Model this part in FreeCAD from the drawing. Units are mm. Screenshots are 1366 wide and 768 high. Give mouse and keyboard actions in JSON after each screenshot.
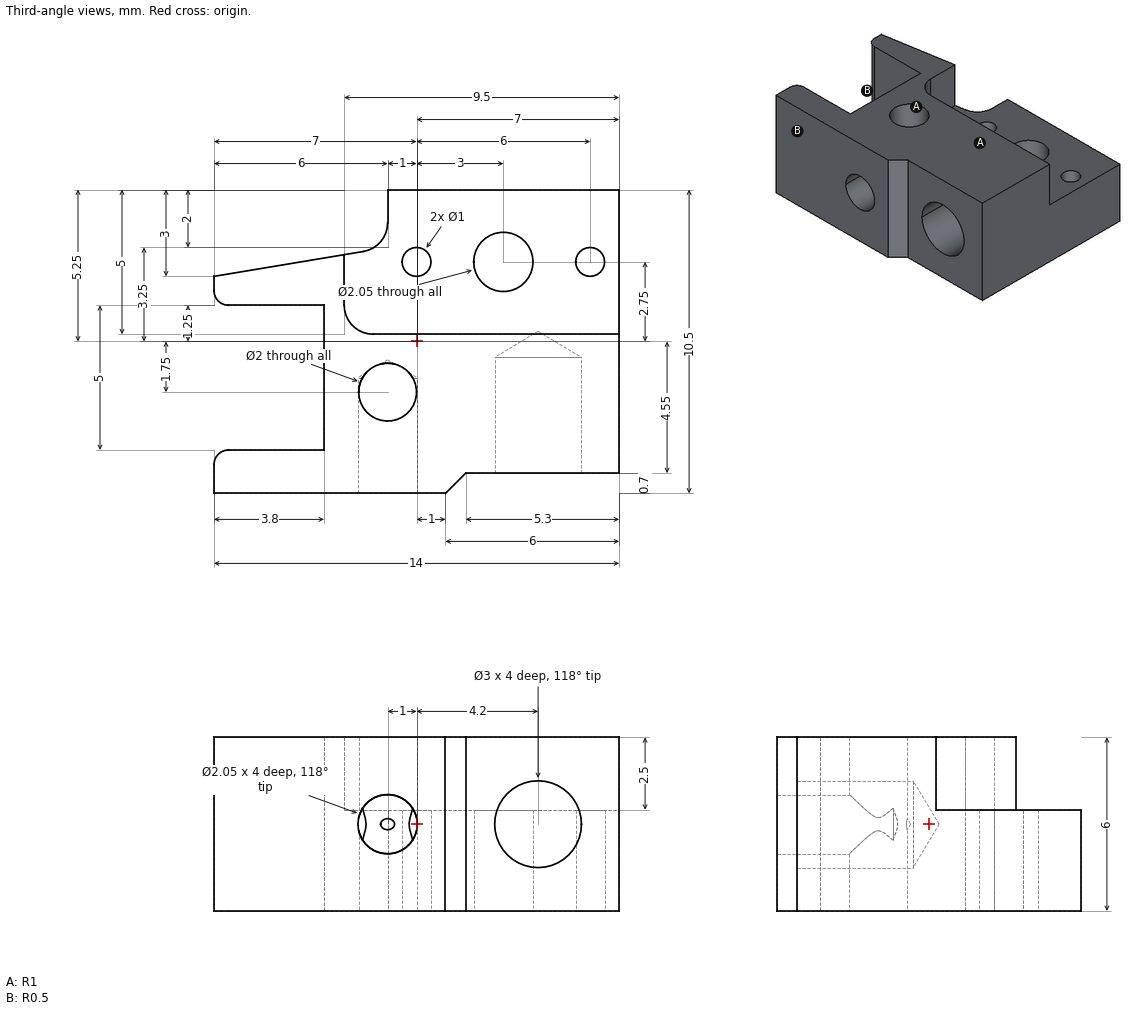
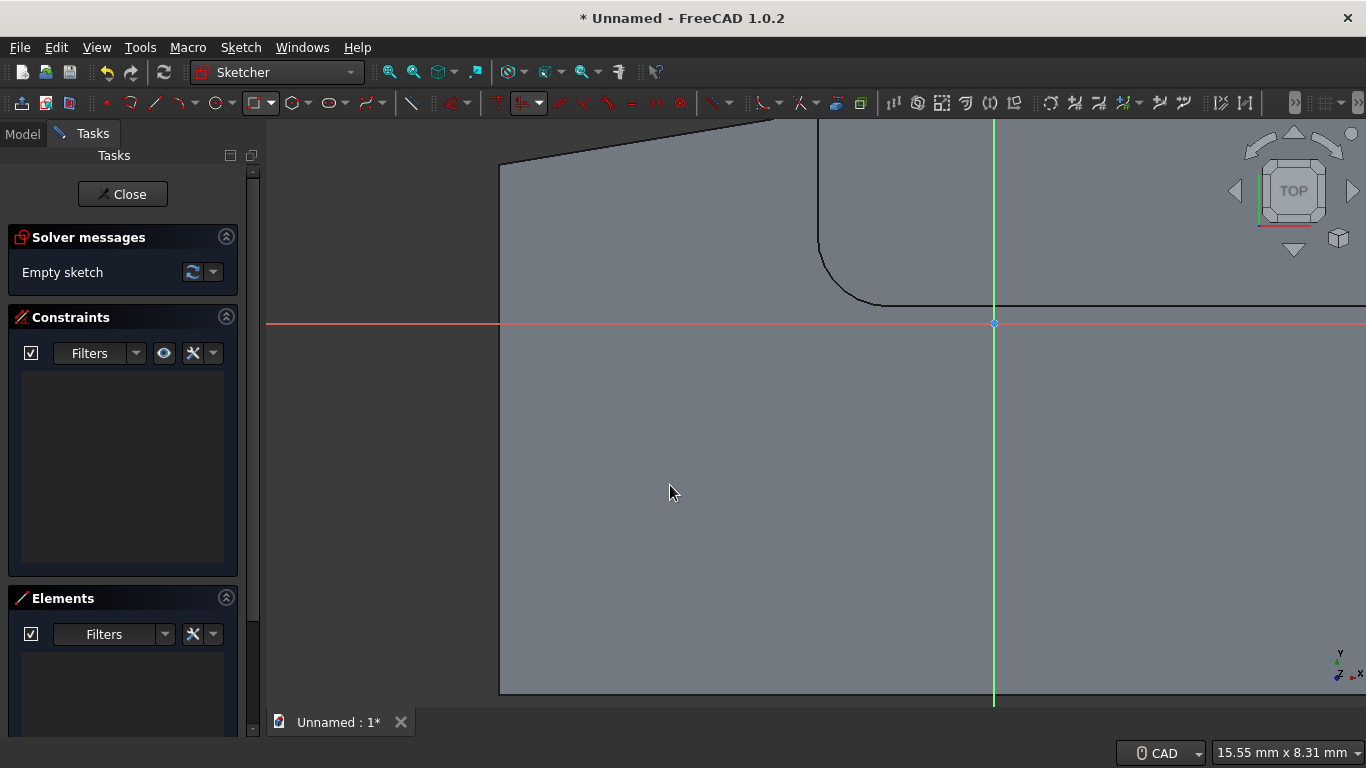
{"action": "left_click", "coordinate": [254, 104]}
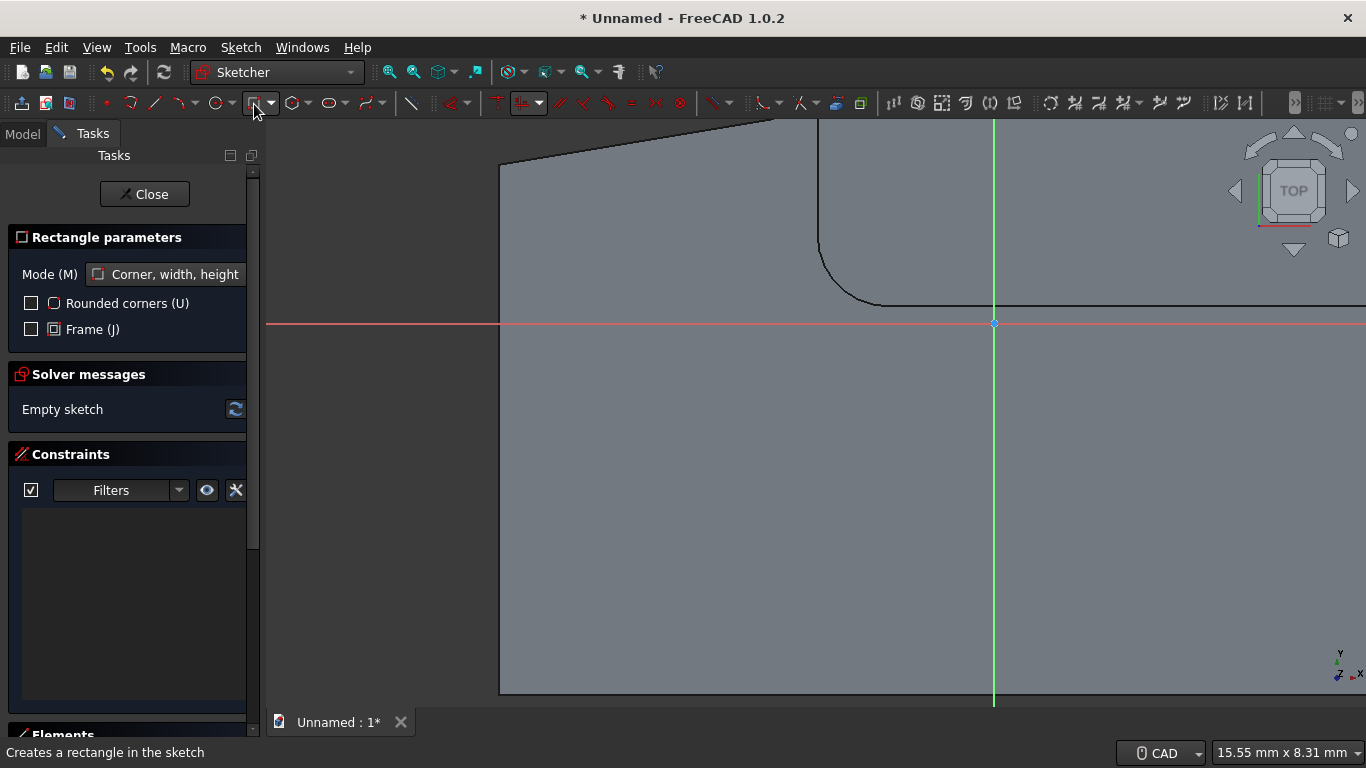
{"action": "left_click", "coordinate": [499, 236]}
{"action": "left_click", "coordinate": [768, 589]}
{"action": "key", "text": "Escape"}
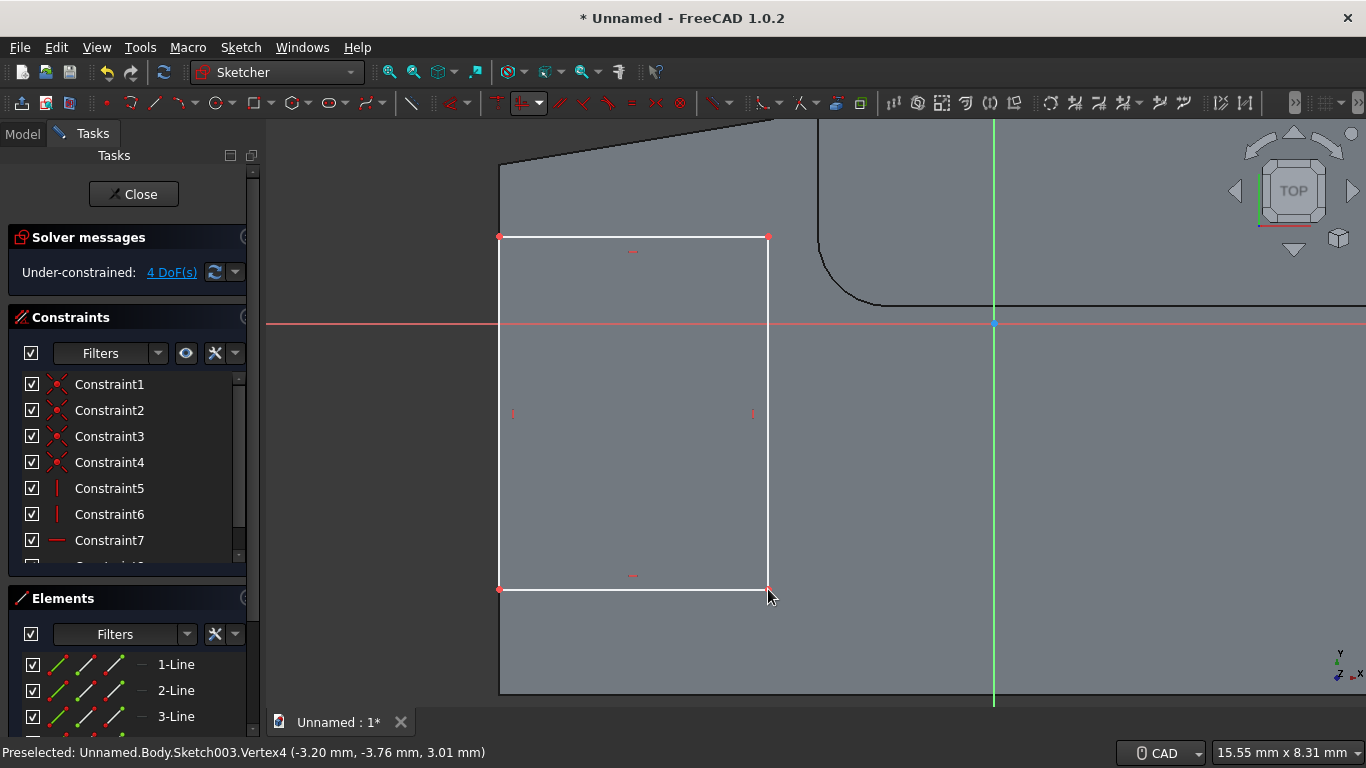
{"action": "left_click", "coordinate": [450, 104]}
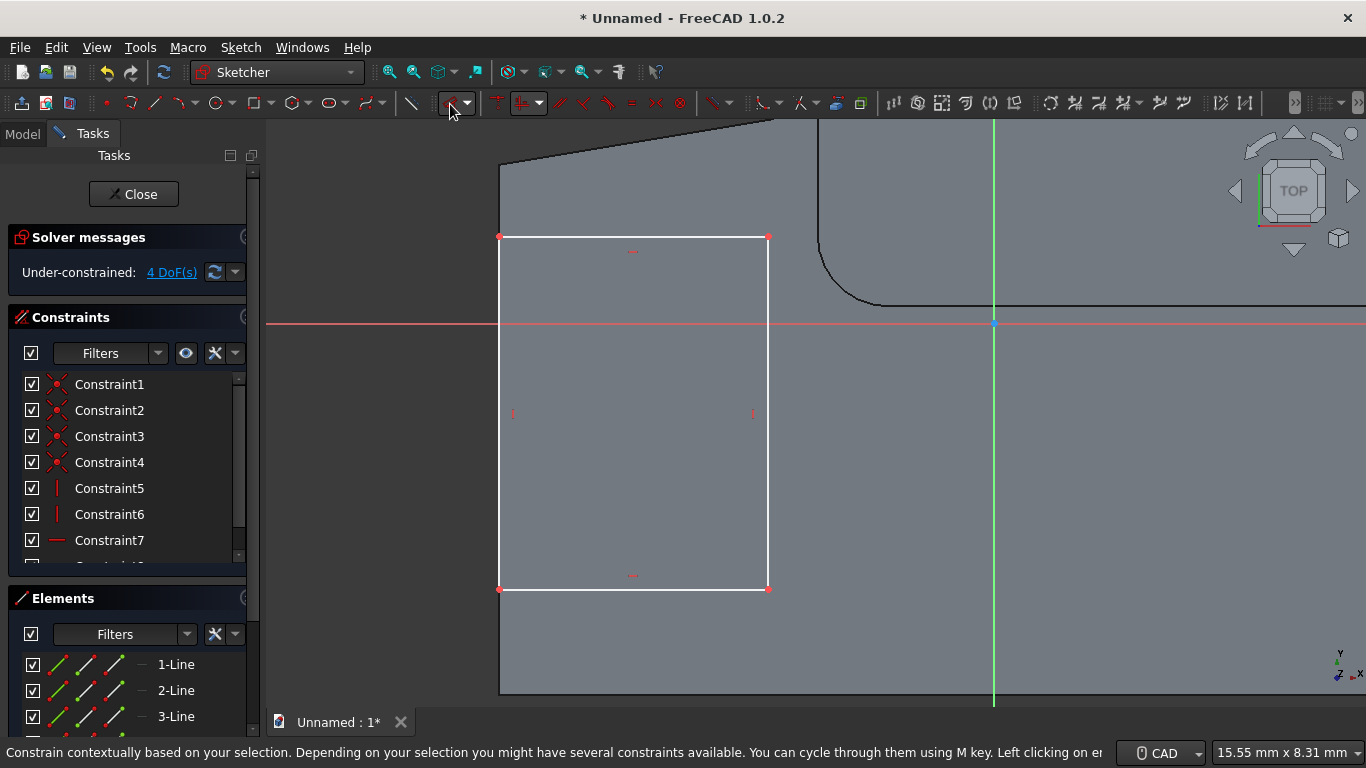
{"action": "left_click", "coordinate": [499, 343]}
{"action": "left_click", "coordinate": [465, 414]}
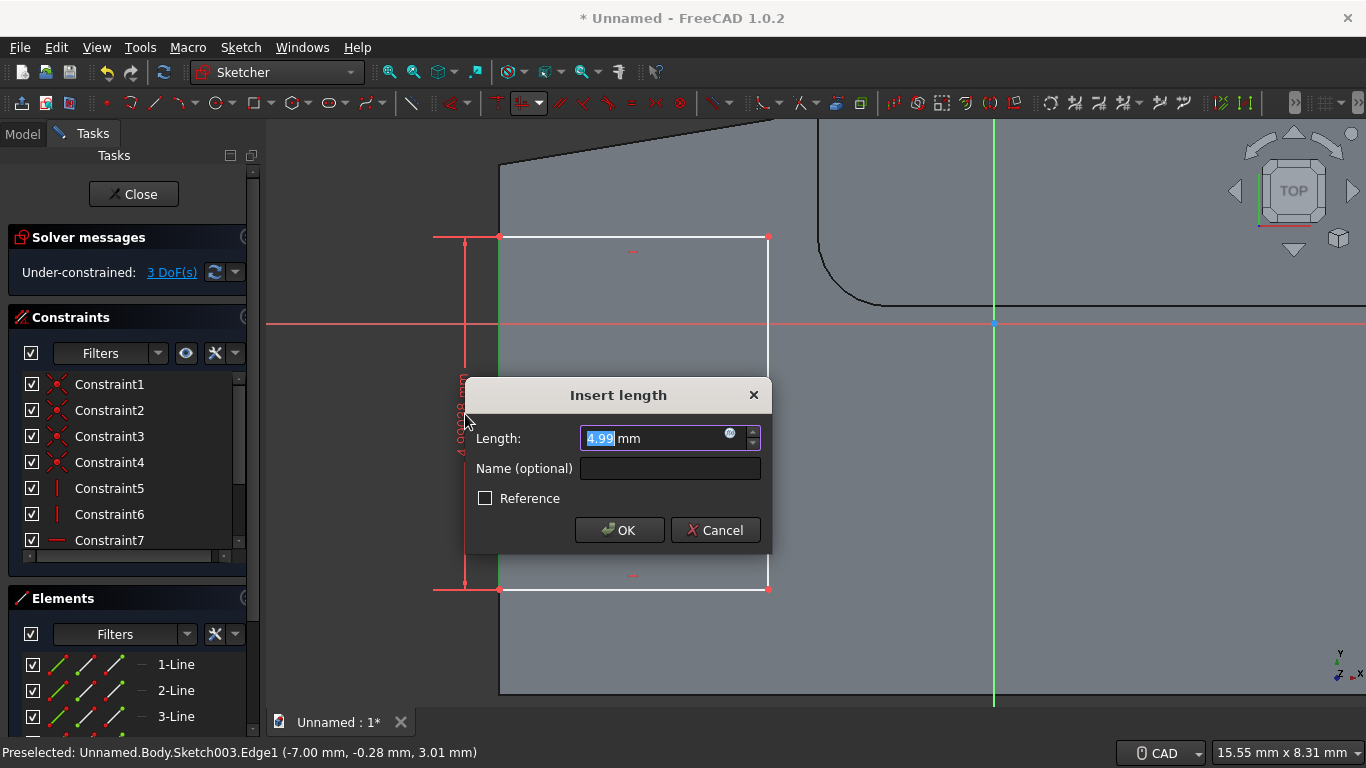
{"action": "type", "text": "5"}
{"action": "key", "text": "Return"}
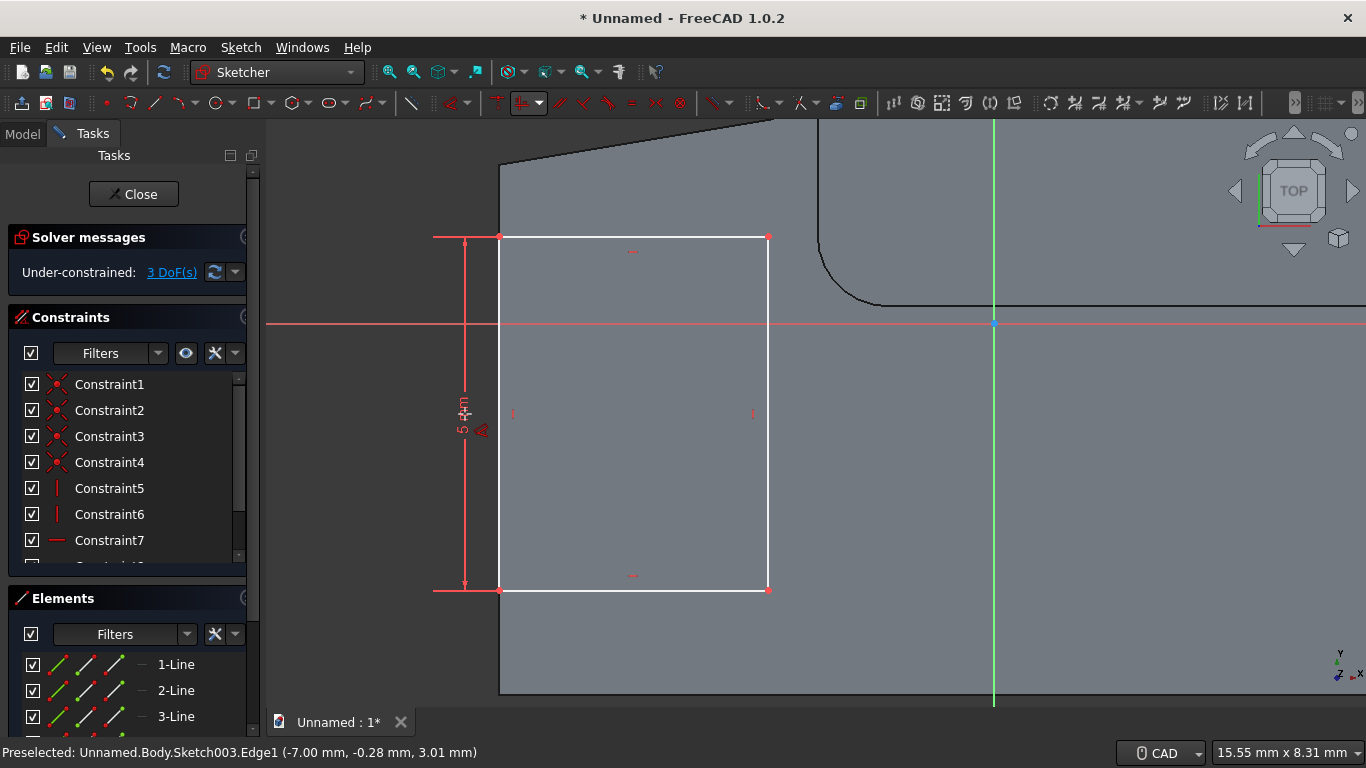
{"action": "left_click", "coordinate": [499, 237]}
{"action": "left_click", "coordinate": [747, 203]}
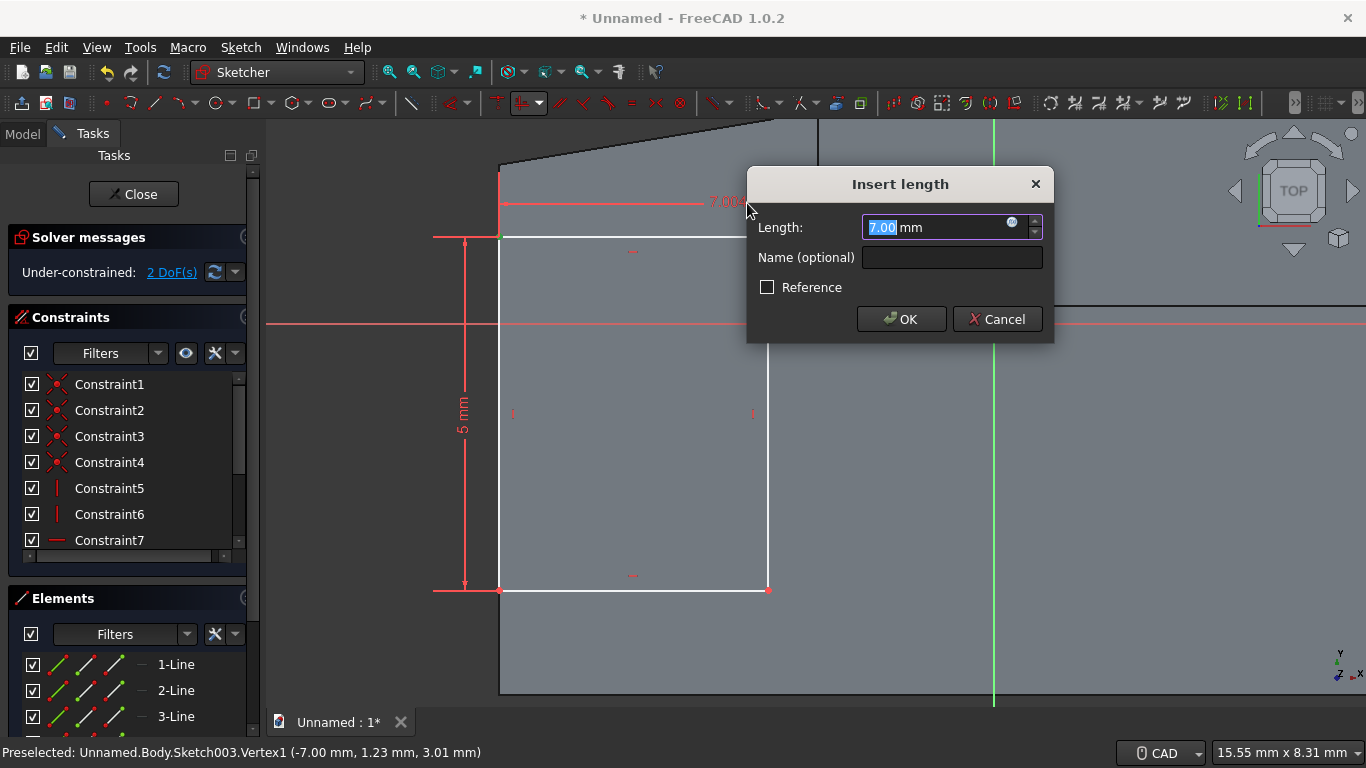
{"action": "type", "text": "7"}
{"action": "key", "text": "Return"}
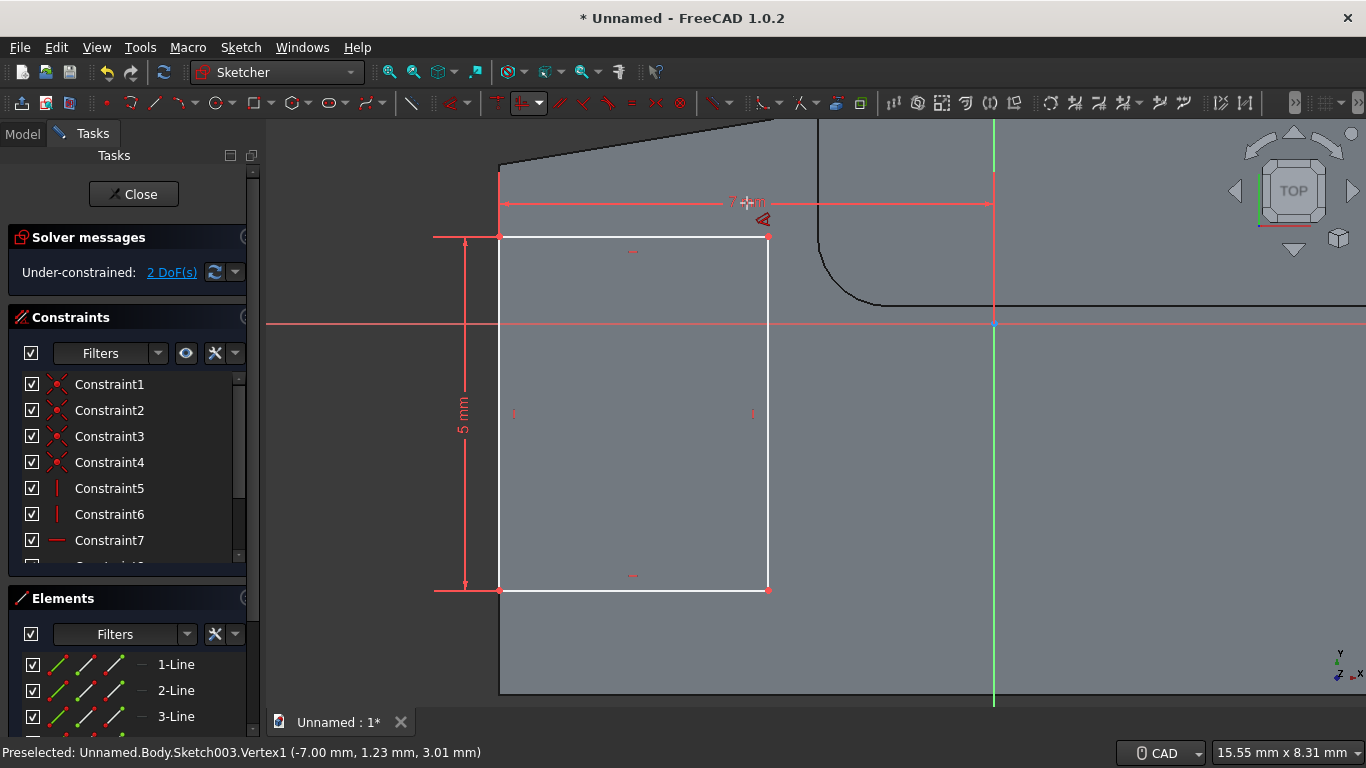
{"action": "left_click", "coordinate": [580, 591]}
{"action": "left_click", "coordinate": [634, 625]}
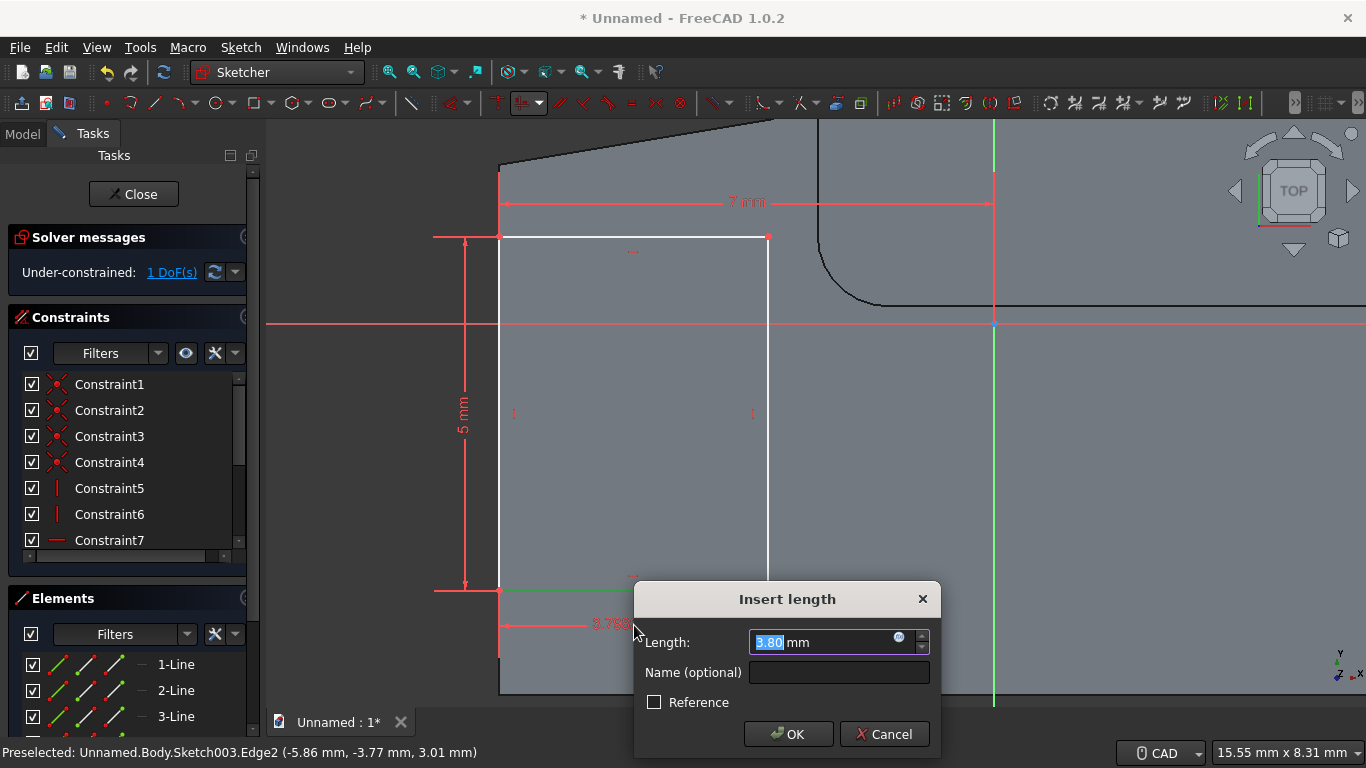
{"action": "type", "text": "3.8"}
{"action": "key", "text": "Return"}